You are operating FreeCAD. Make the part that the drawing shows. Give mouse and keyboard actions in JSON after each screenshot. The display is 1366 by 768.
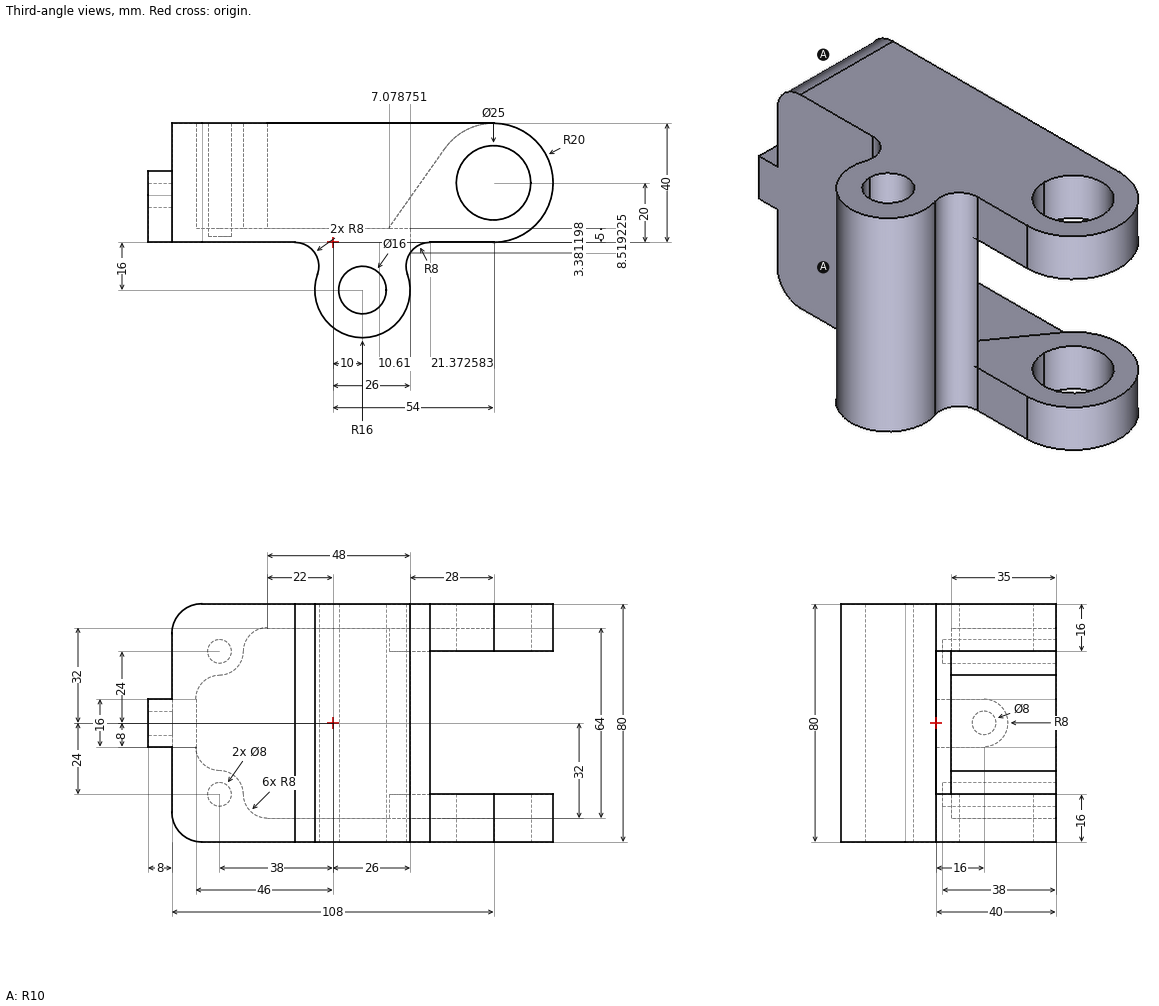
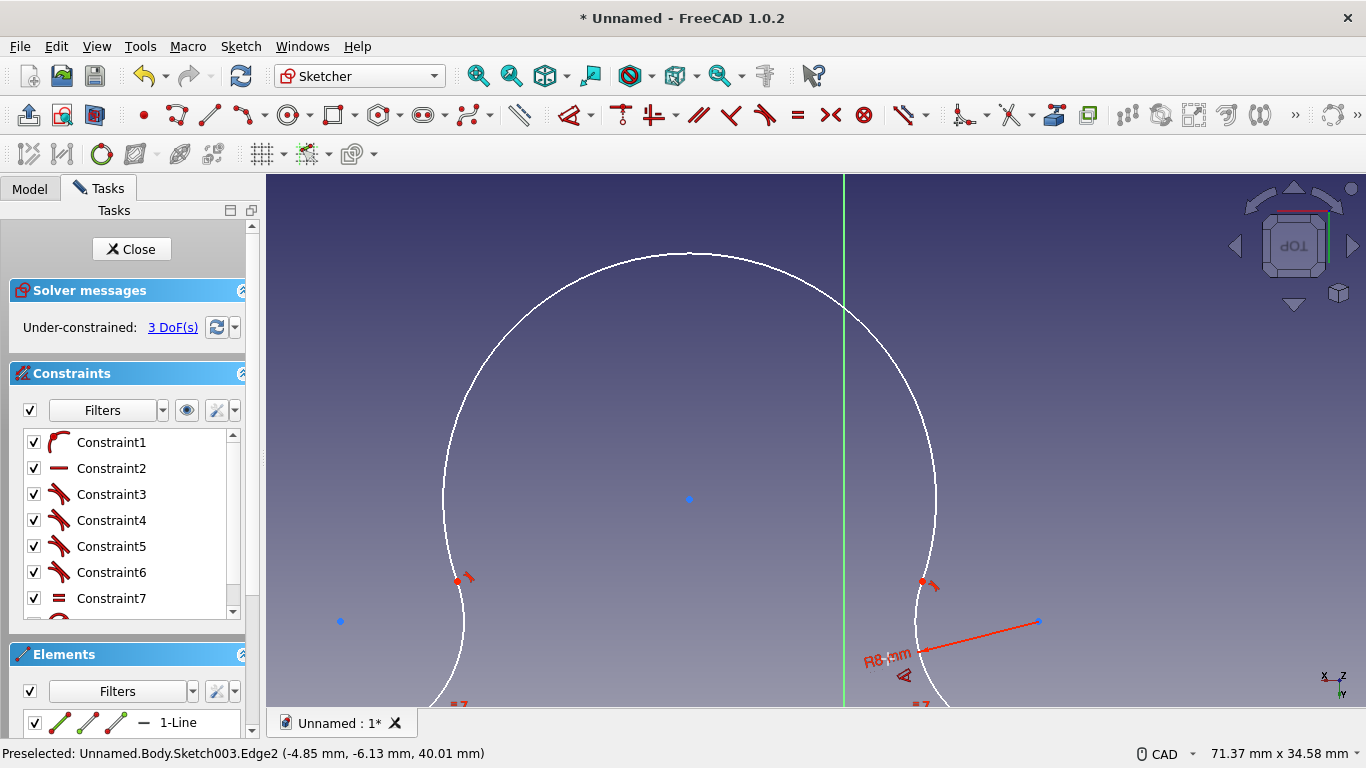
{"action": "left_click", "coordinate": [860, 322]}
{"action": "left_click", "coordinate": [882, 299]}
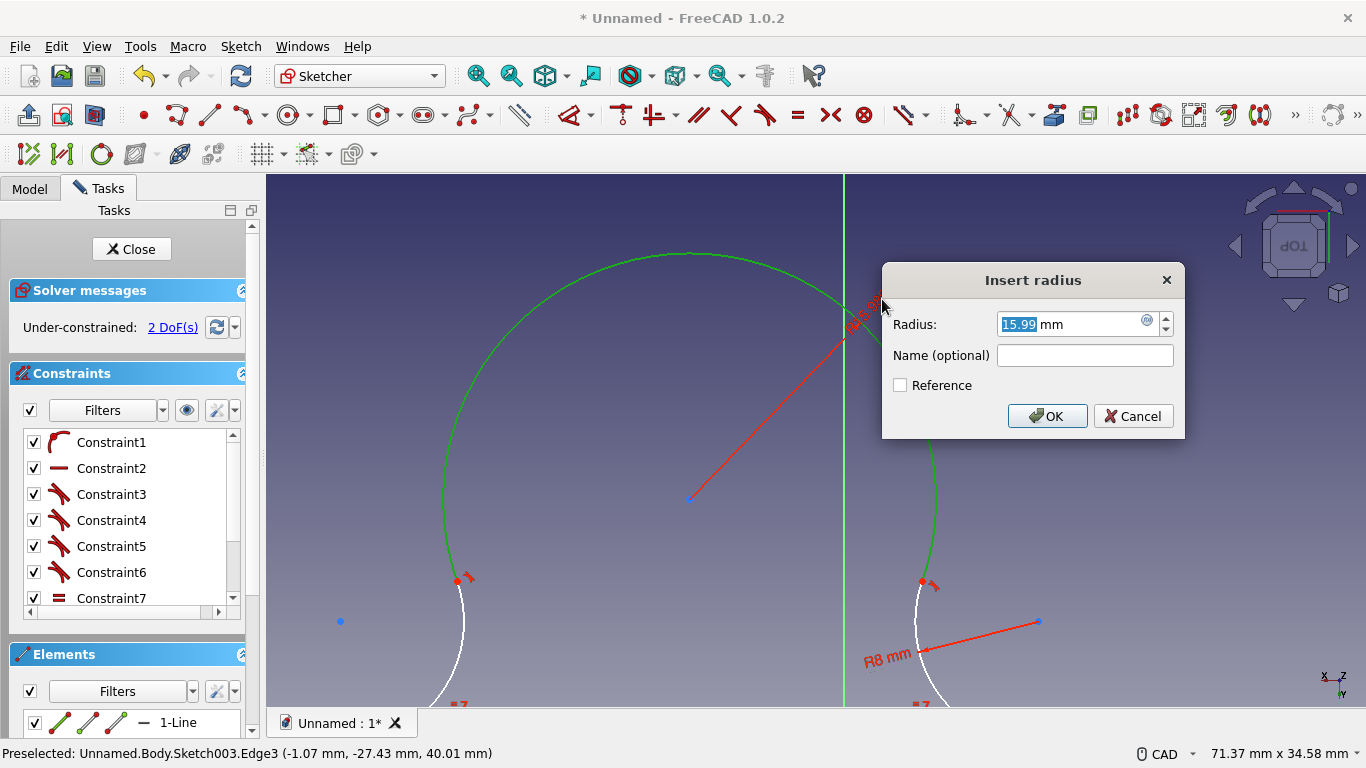
{"action": "type", "text": "16"}
{"action": "key", "text": "Return"}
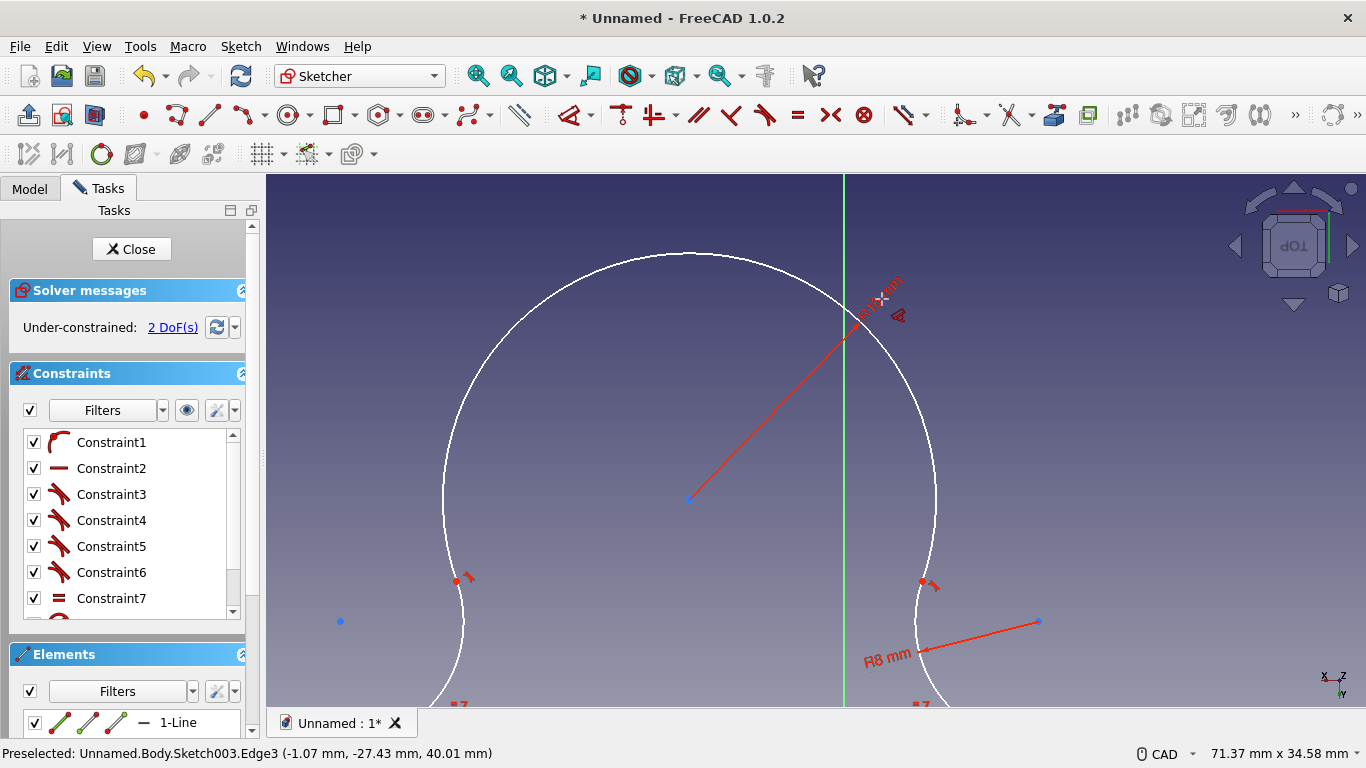
{"action": "left_click", "coordinate": [690, 500]}
{"action": "left_click", "coordinate": [767, 466]}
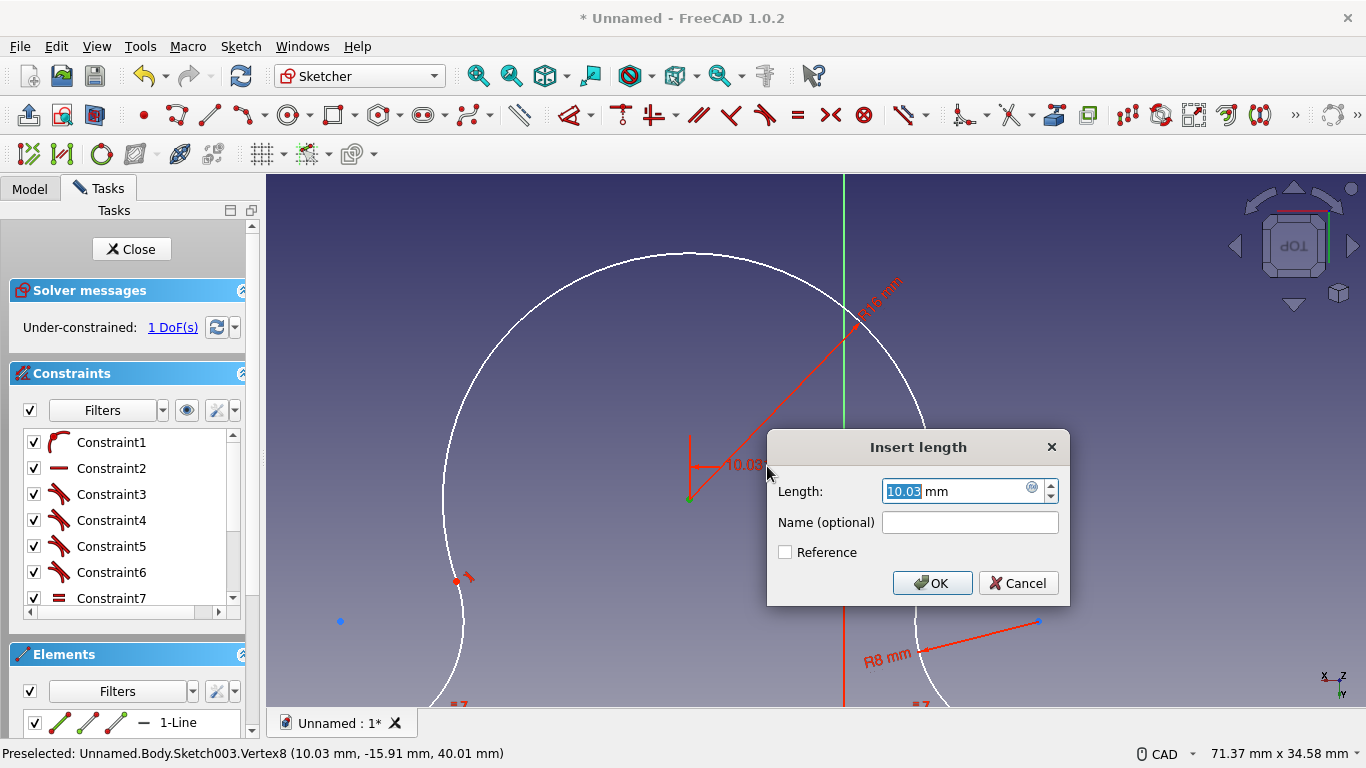
{"action": "type", "text": "10"}
{"action": "key", "text": "Return"}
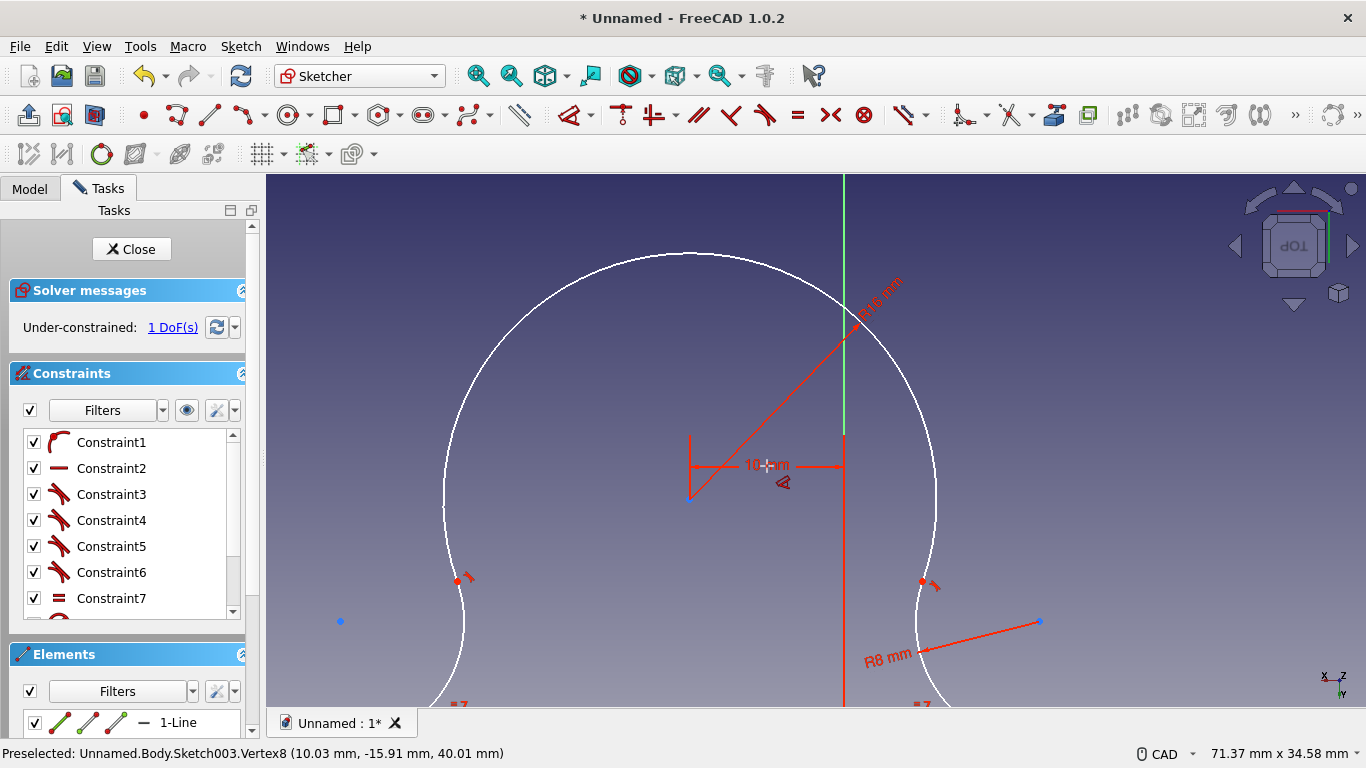
{"action": "left_click", "coordinate": [690, 500]}
{"action": "left_click", "coordinate": [878, 589]}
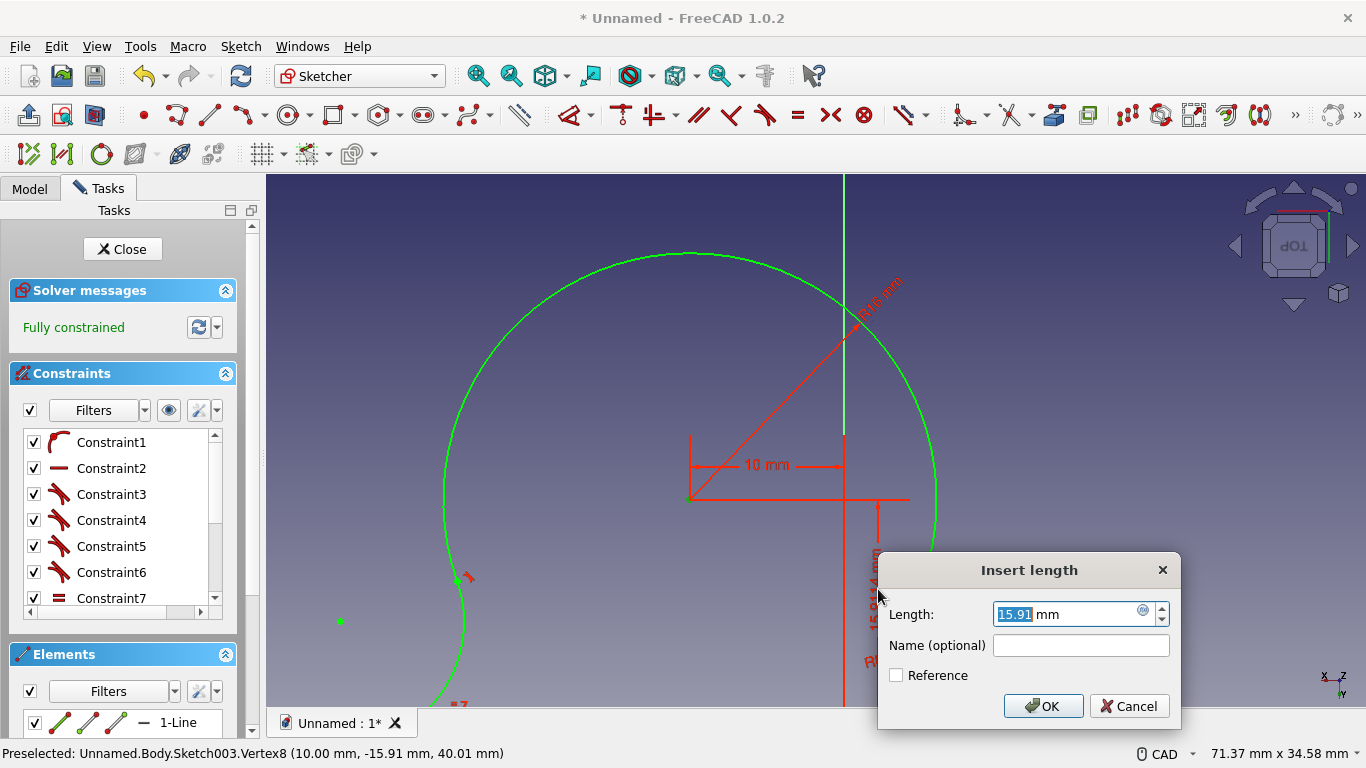
{"action": "type", "text": "16"}
{"action": "key", "text": "Return"}
{"action": "key", "text": "Escape"}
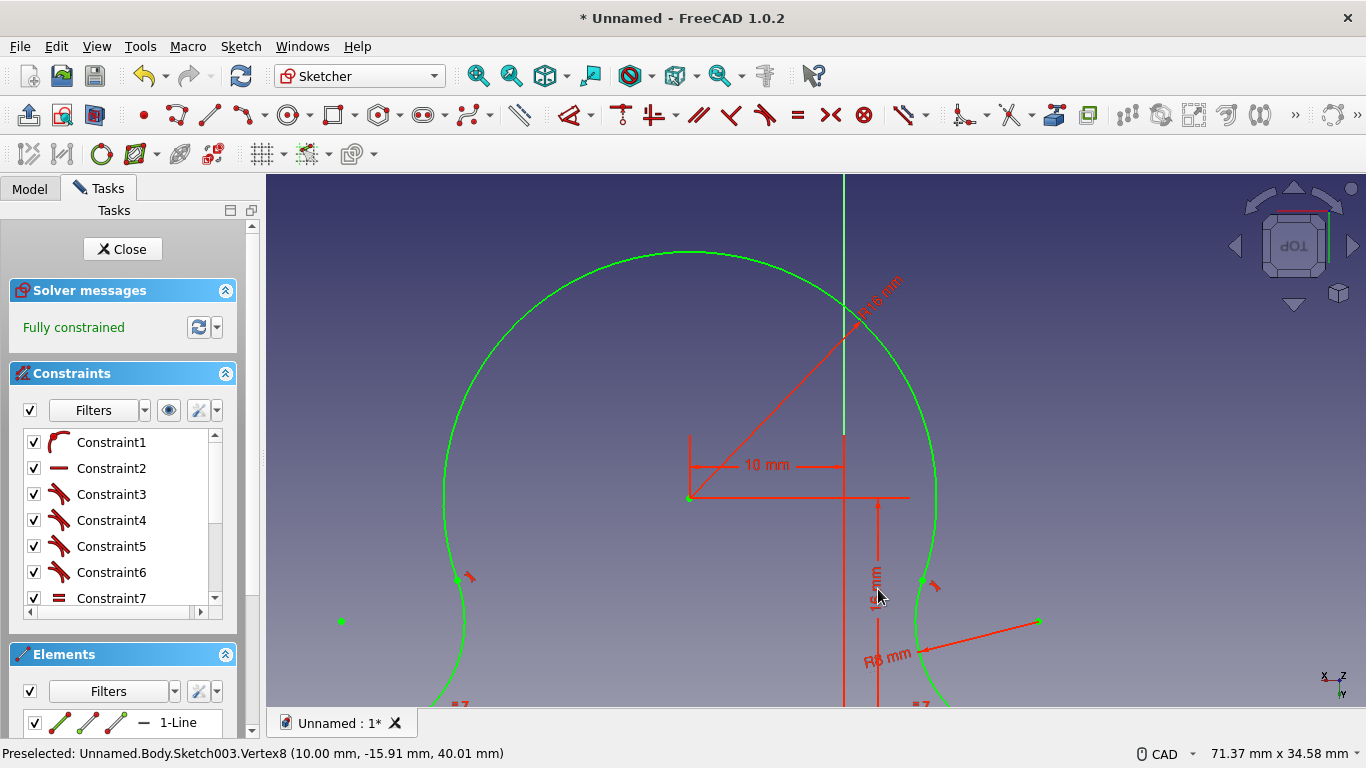
{"action": "left_click", "coordinate": [123, 249]}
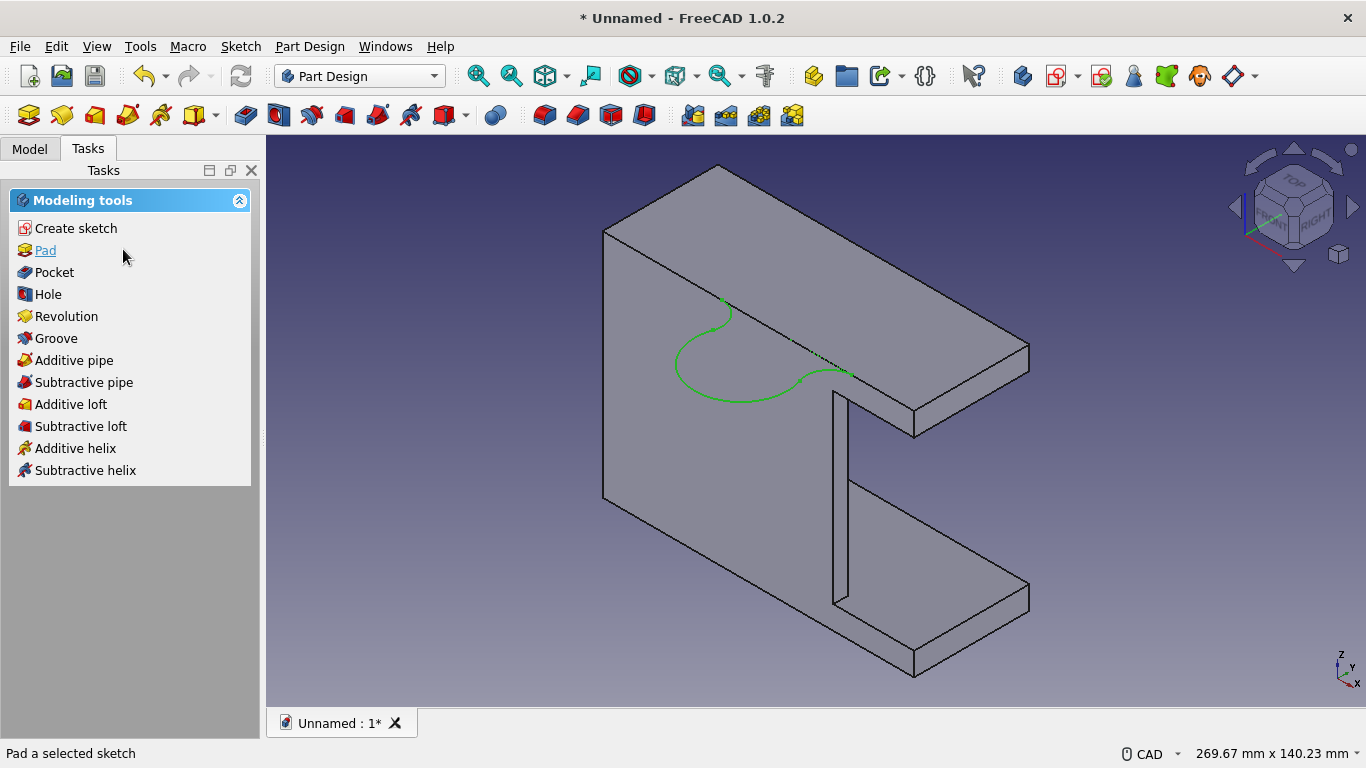
{"action": "left_click", "coordinate": [29, 116]}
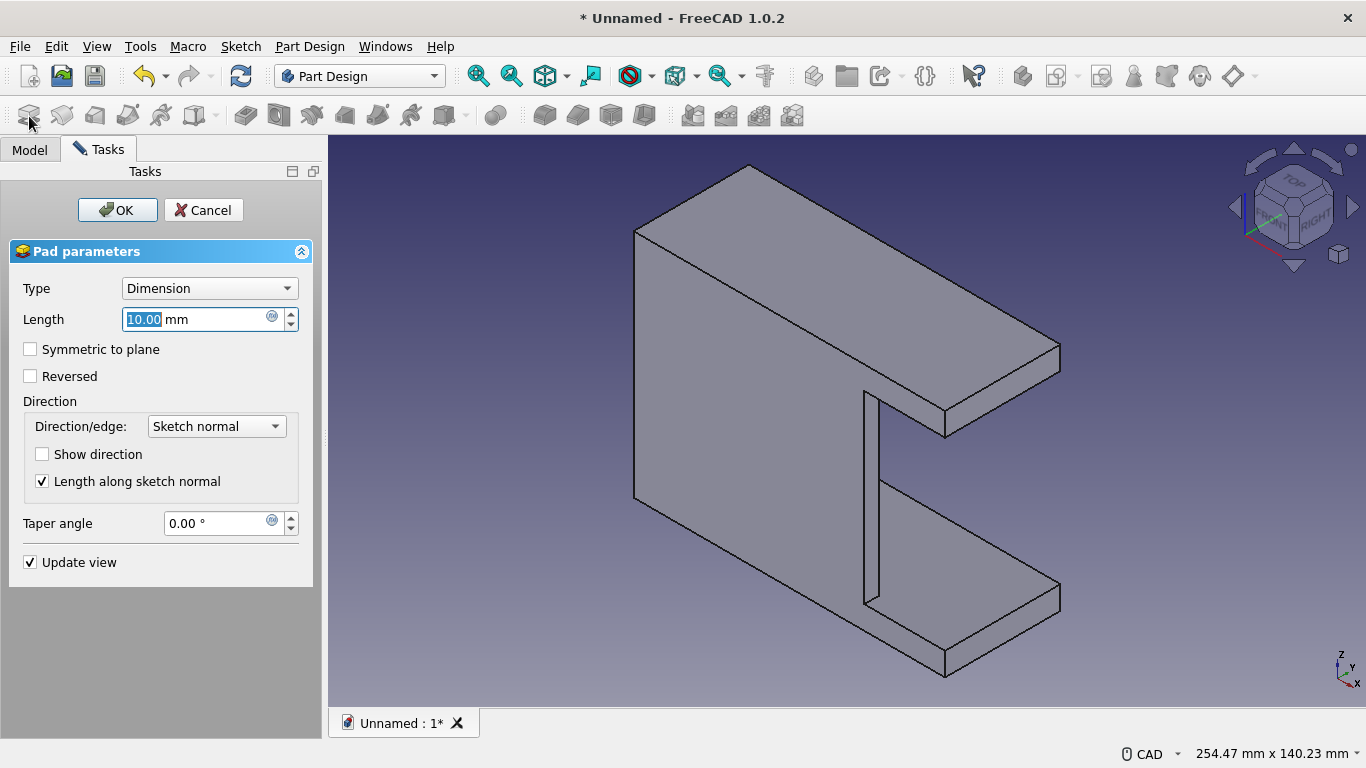
{"action": "type", "text": "80"}
{"action": "key", "text": "Tab"}